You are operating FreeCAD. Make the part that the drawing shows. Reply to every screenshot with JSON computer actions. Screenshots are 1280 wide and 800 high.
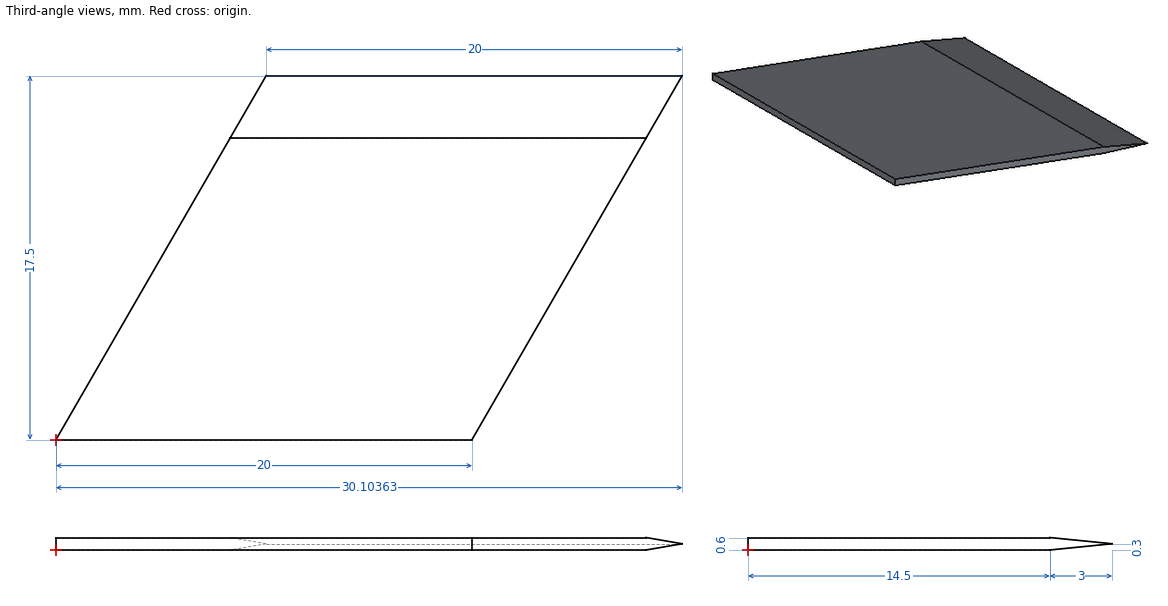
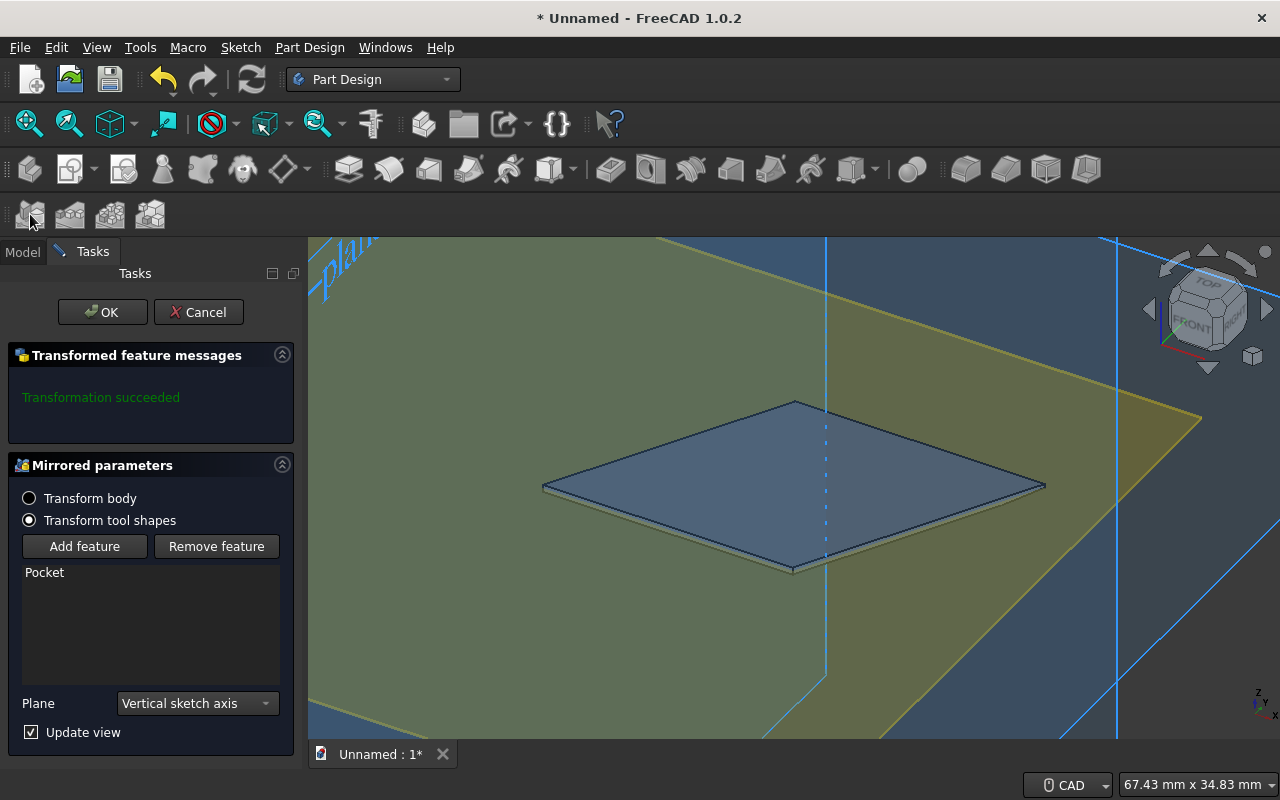
{"action": "left_click", "coordinate": [198, 704]}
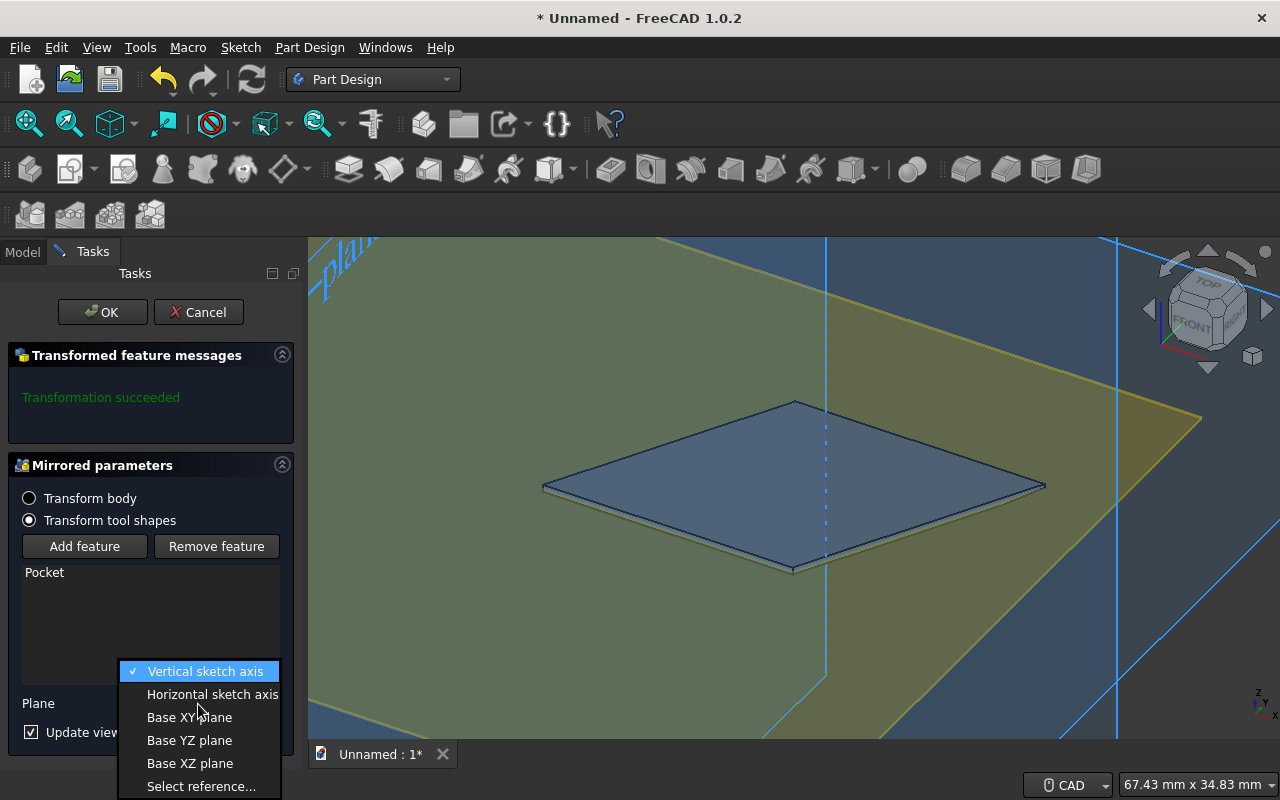
{"action": "left_click", "coordinate": [198, 786]}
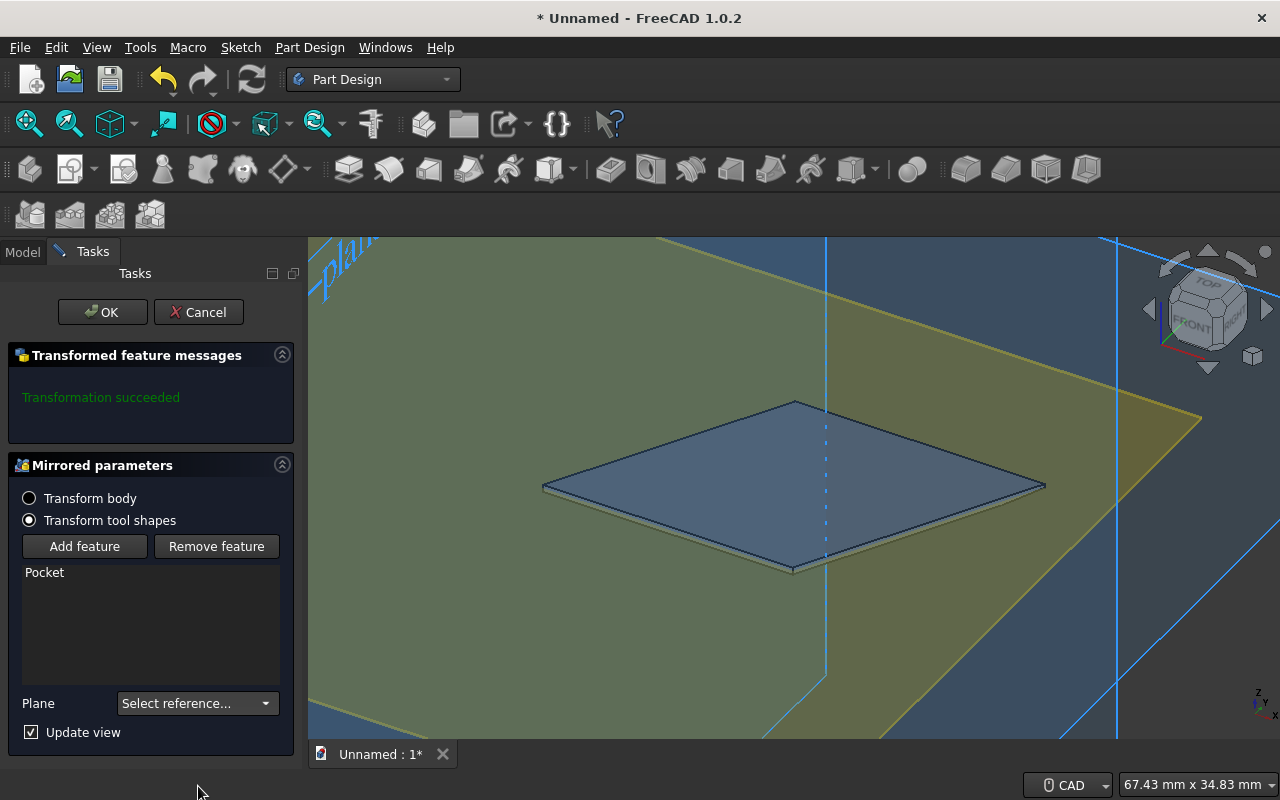
{"action": "left_click", "coordinate": [23, 251]}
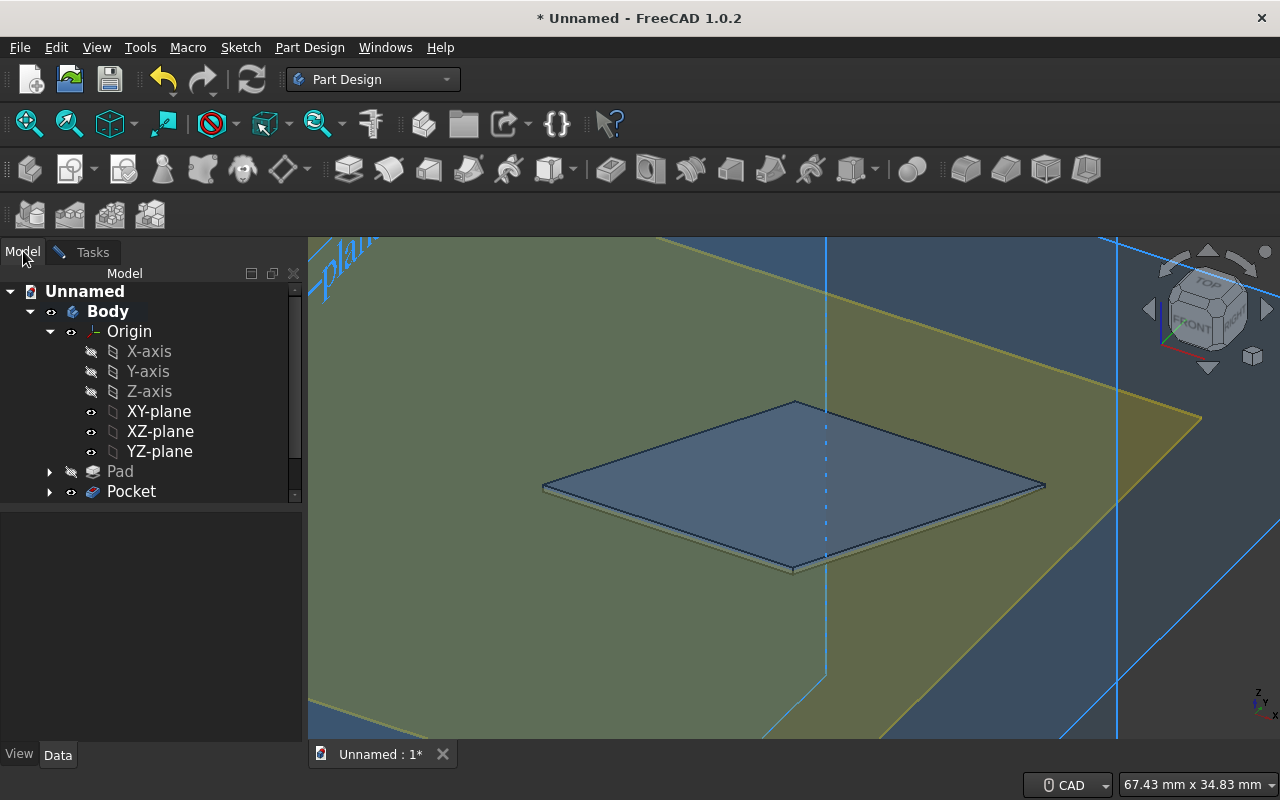
{"action": "scroll", "coordinate": [100, 387], "scroll_direction": "down", "scroll_amount": 3}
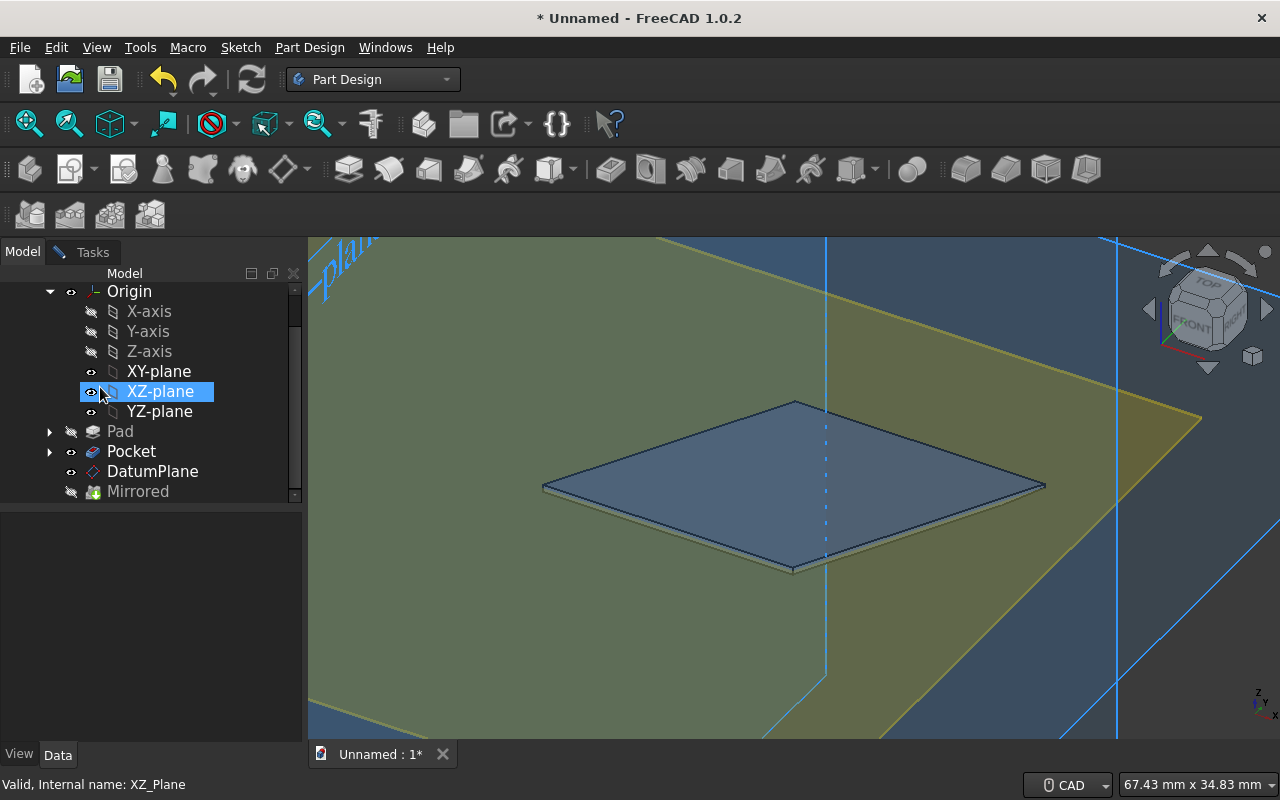
{"action": "left_click", "coordinate": [116, 472]}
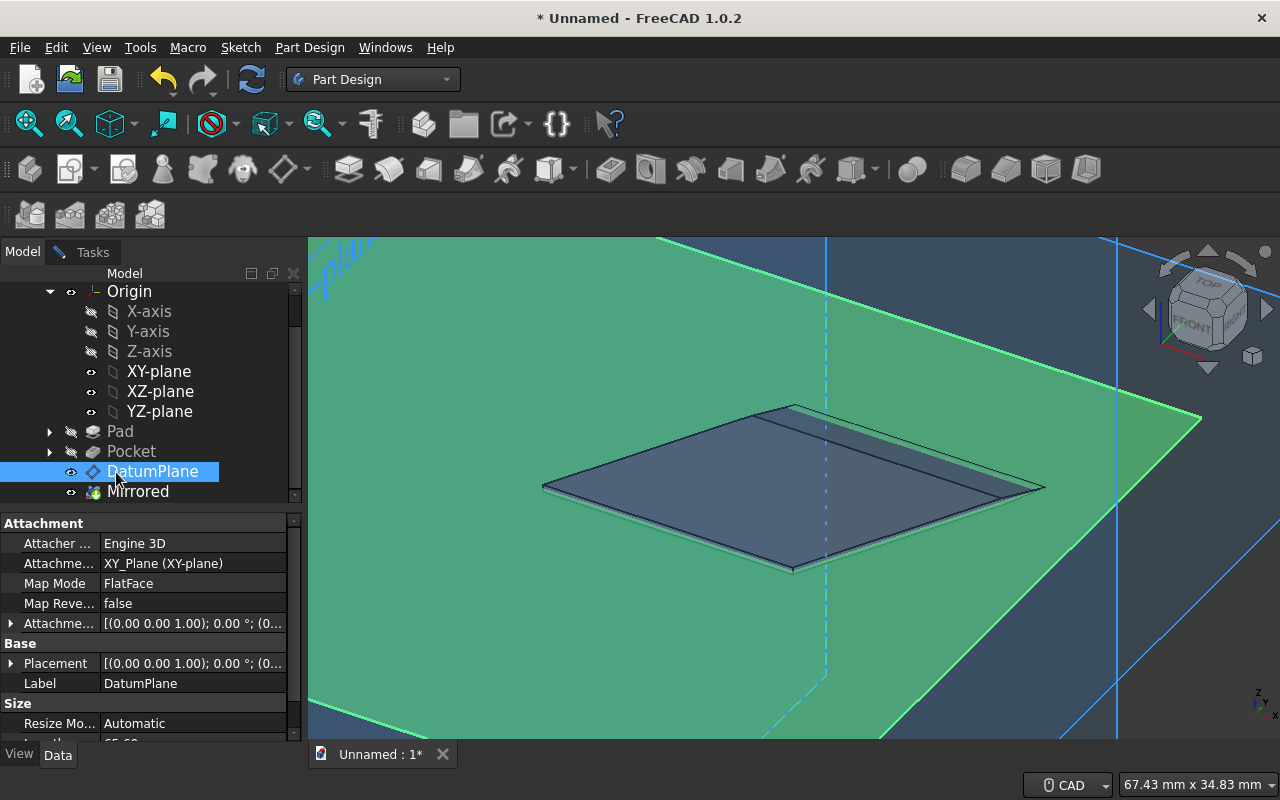
{"action": "left_click", "coordinate": [84, 251]}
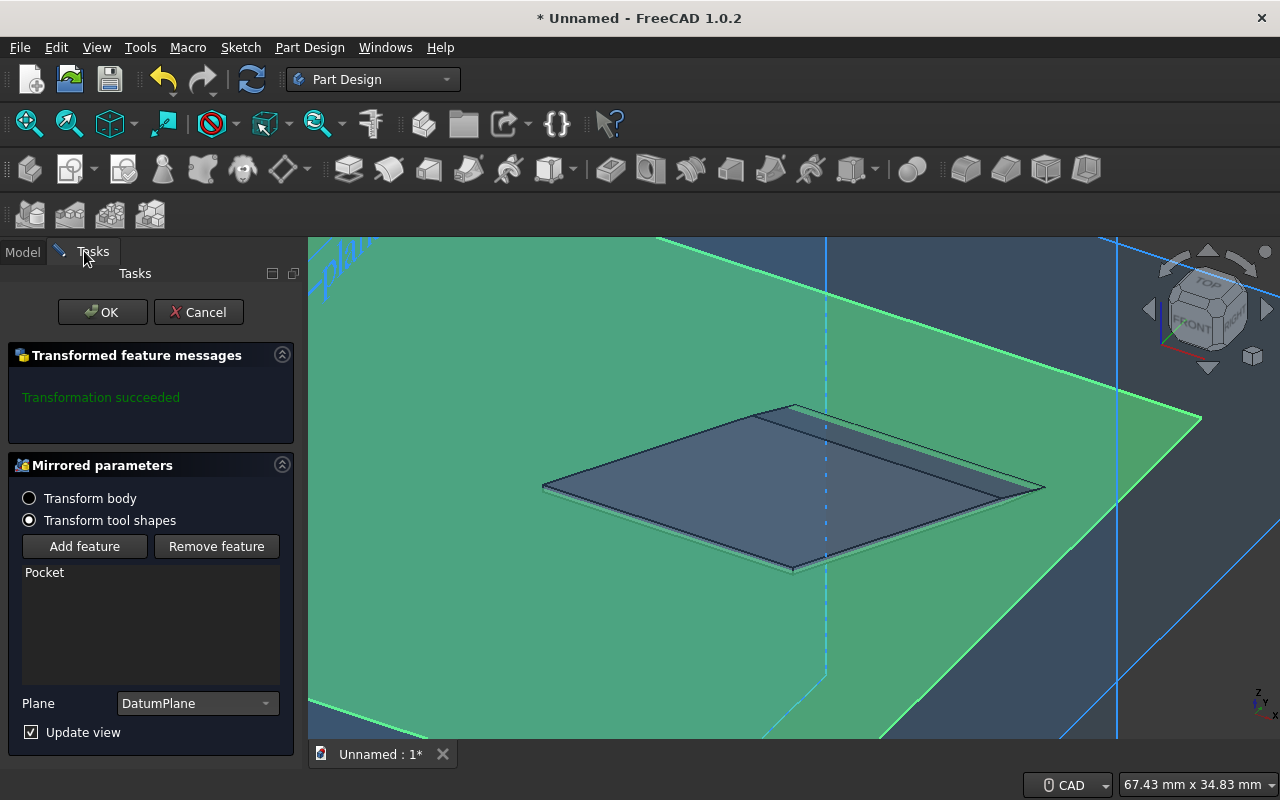
{"action": "left_click", "coordinate": [103, 312]}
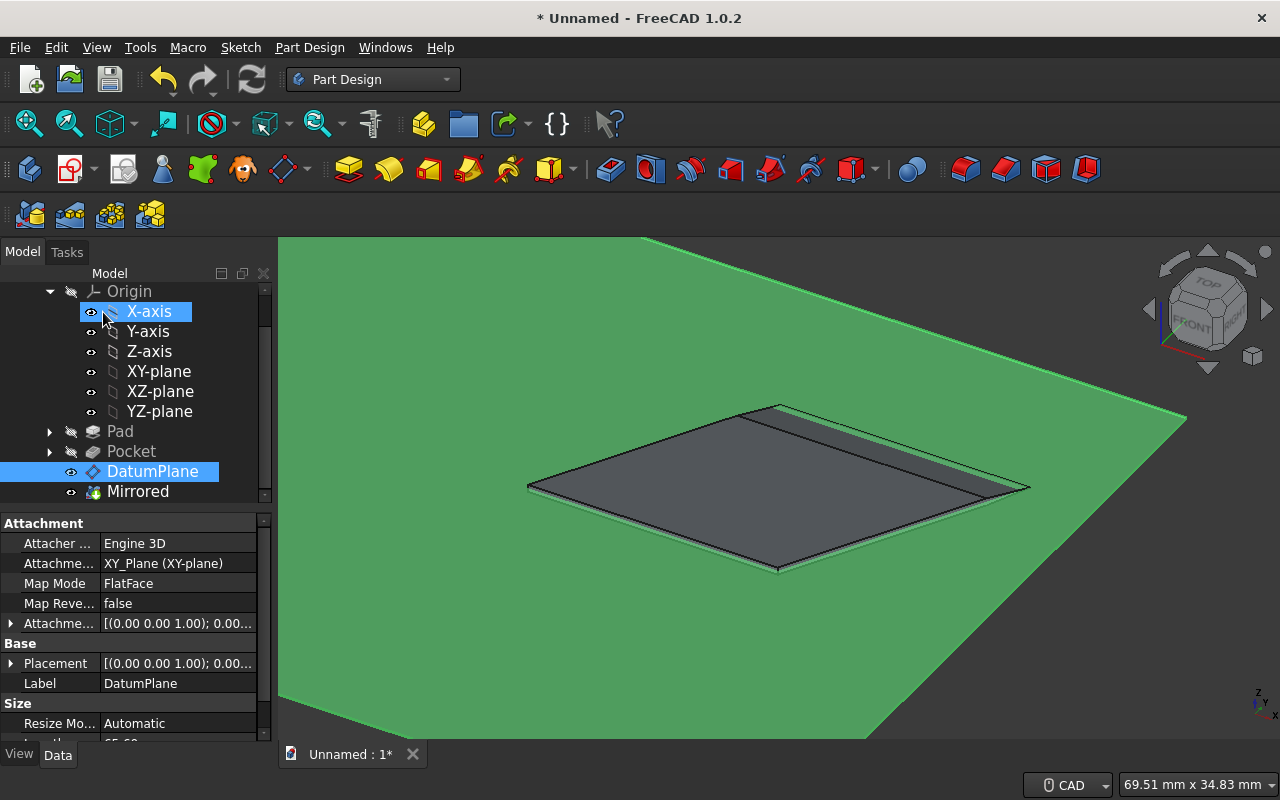
{"action": "left_click", "coordinate": [116, 472]}
{"action": "key", "text": "space"}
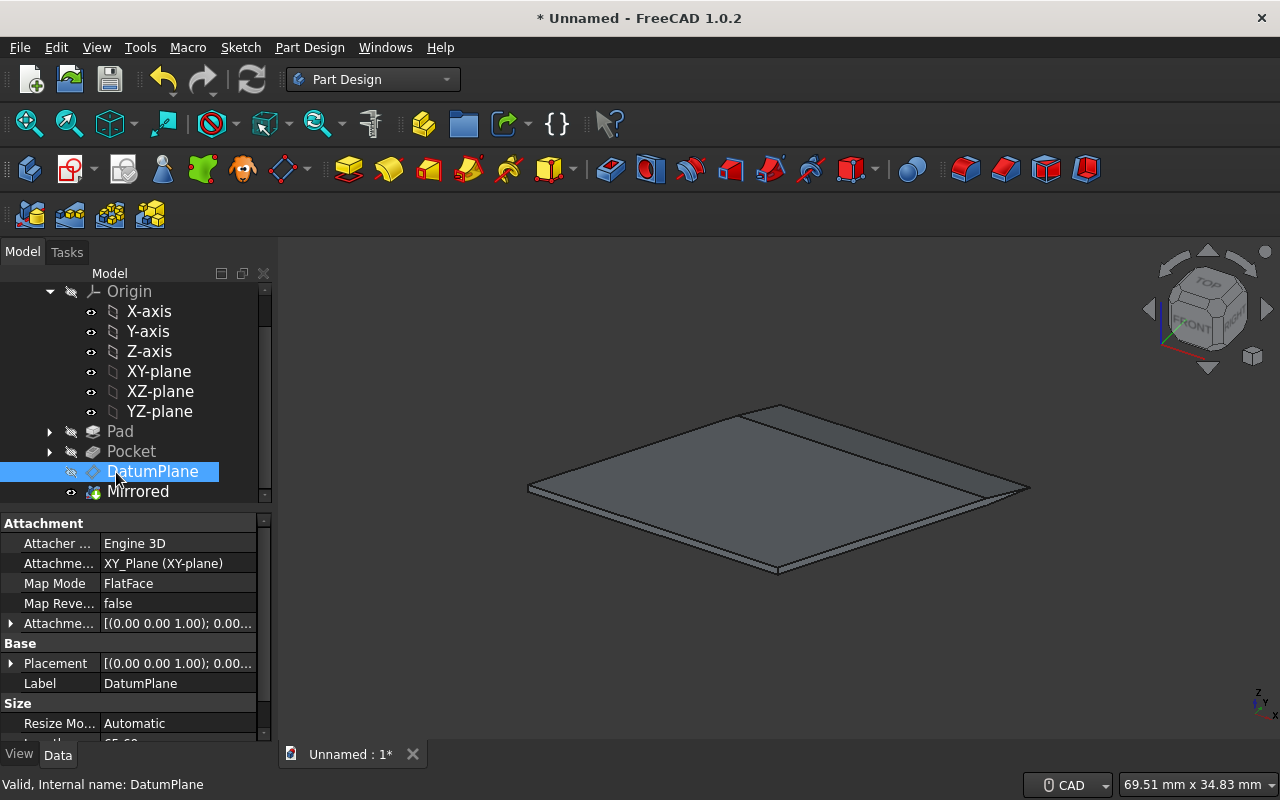
{"action": "key", "text": "0"}